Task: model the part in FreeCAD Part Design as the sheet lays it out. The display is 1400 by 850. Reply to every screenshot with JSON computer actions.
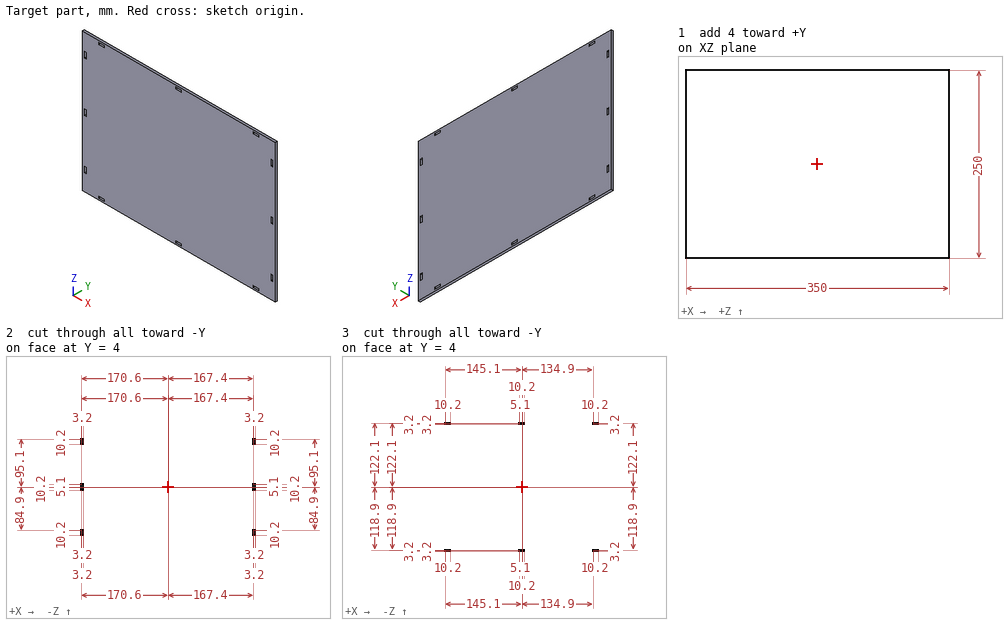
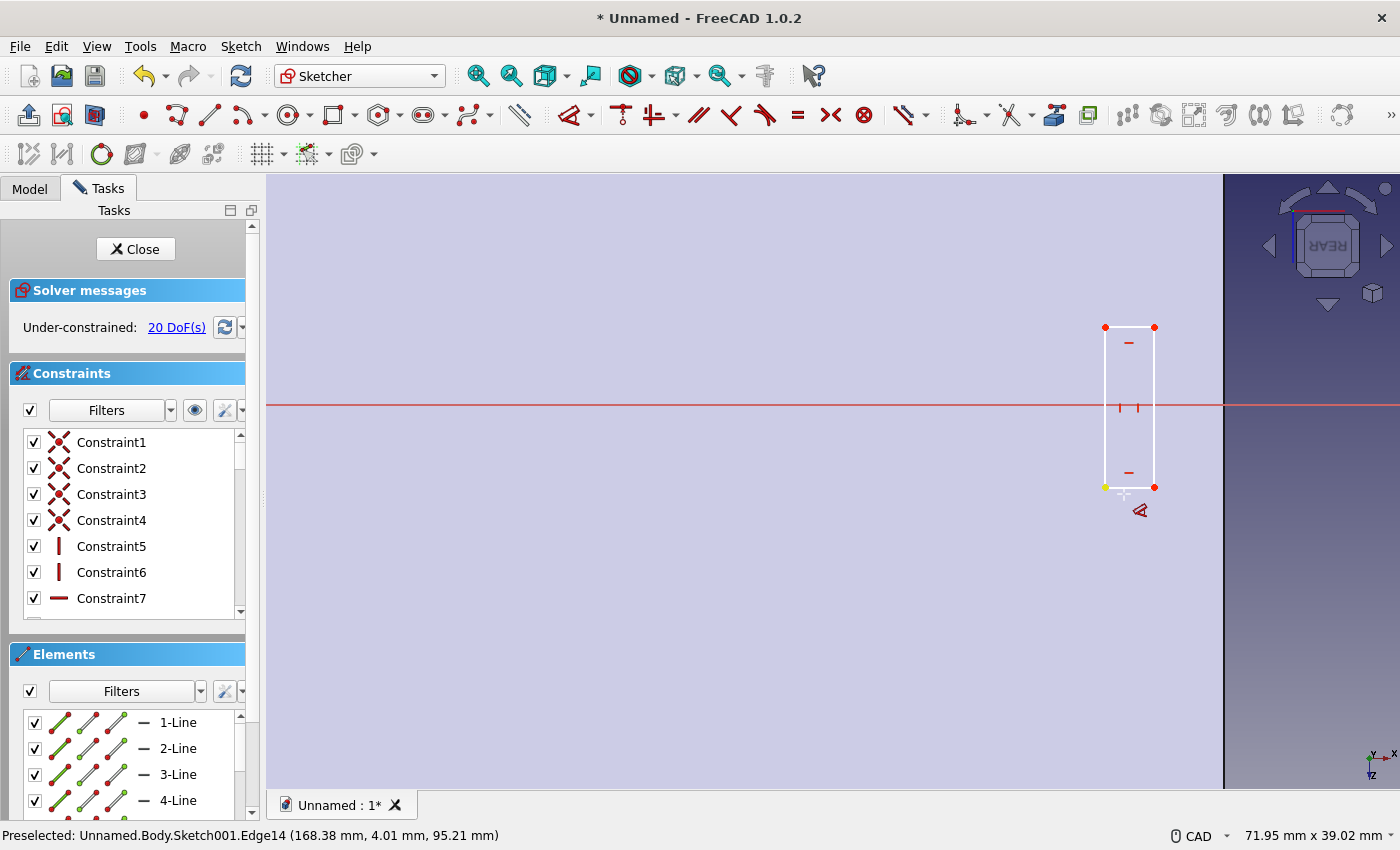
{"action": "left_click", "coordinate": [1120, 488]}
{"action": "left_click", "coordinate": [1130, 522]}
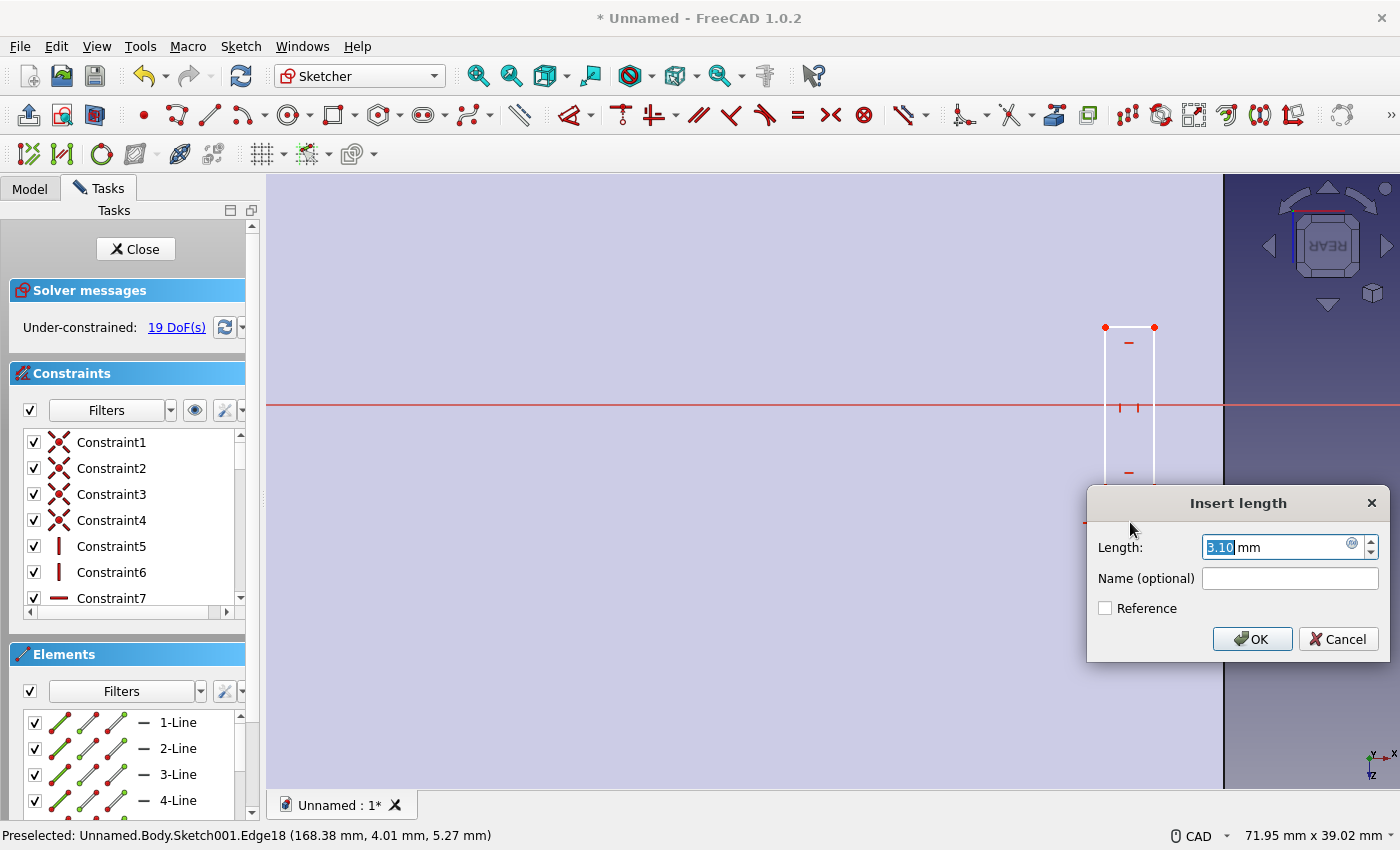
{"action": "type", "text": "3.2"}
{"action": "key", "text": "Return"}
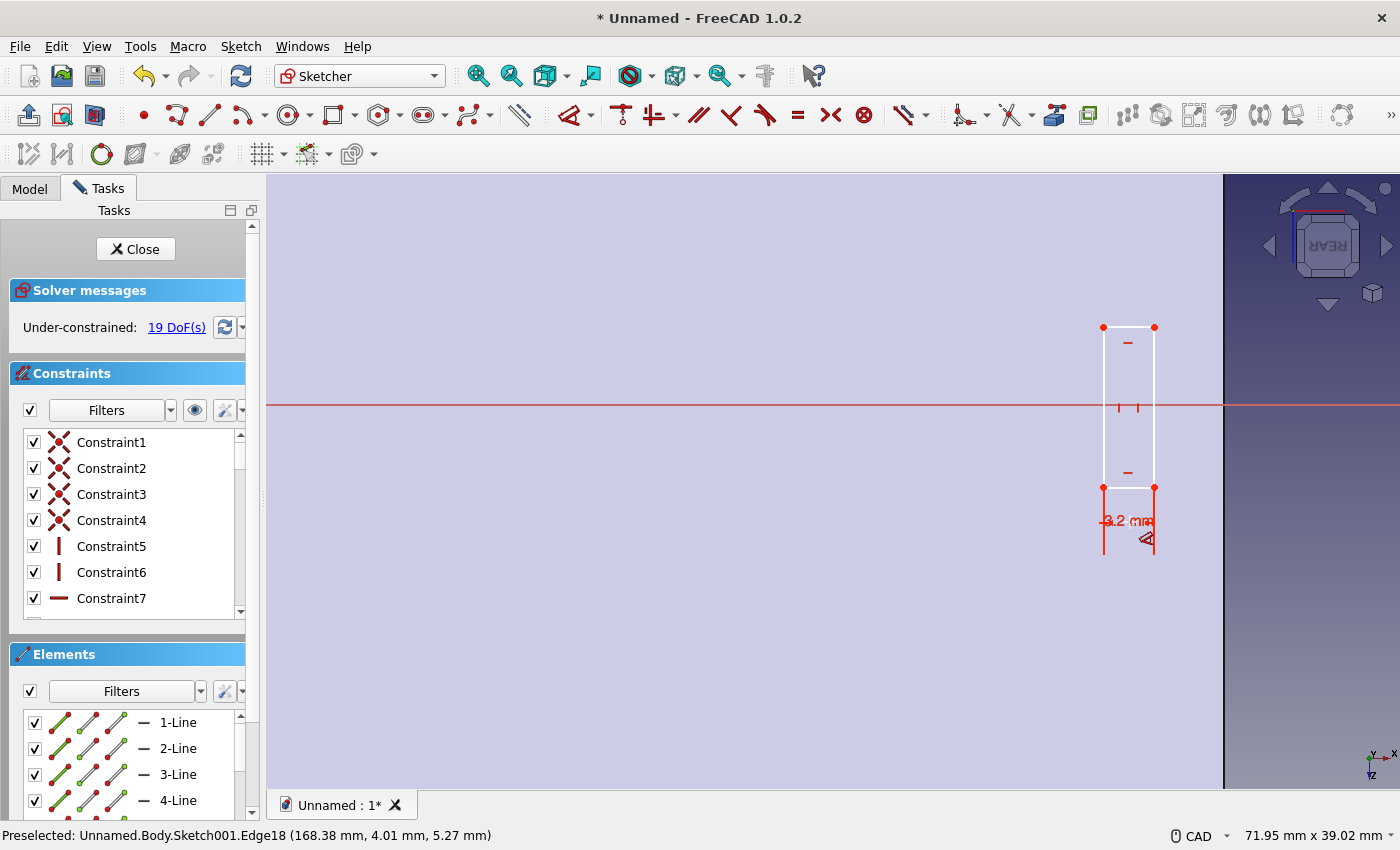
{"action": "scroll", "coordinate": [1124, 494], "scroll_direction": "down", "scroll_amount": 10}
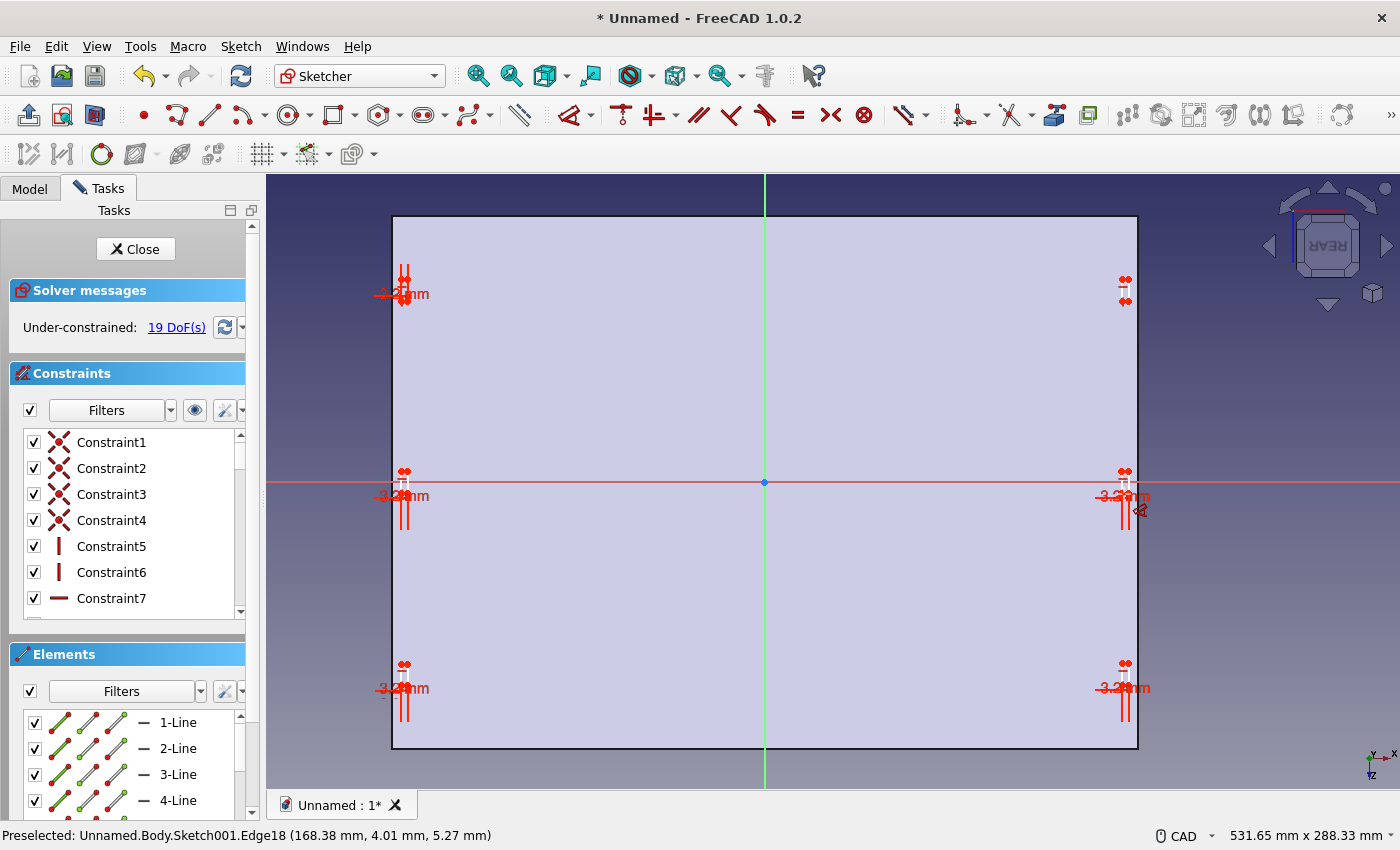
{"action": "scroll", "coordinate": [1124, 302], "scroll_direction": "up", "scroll_amount": 10}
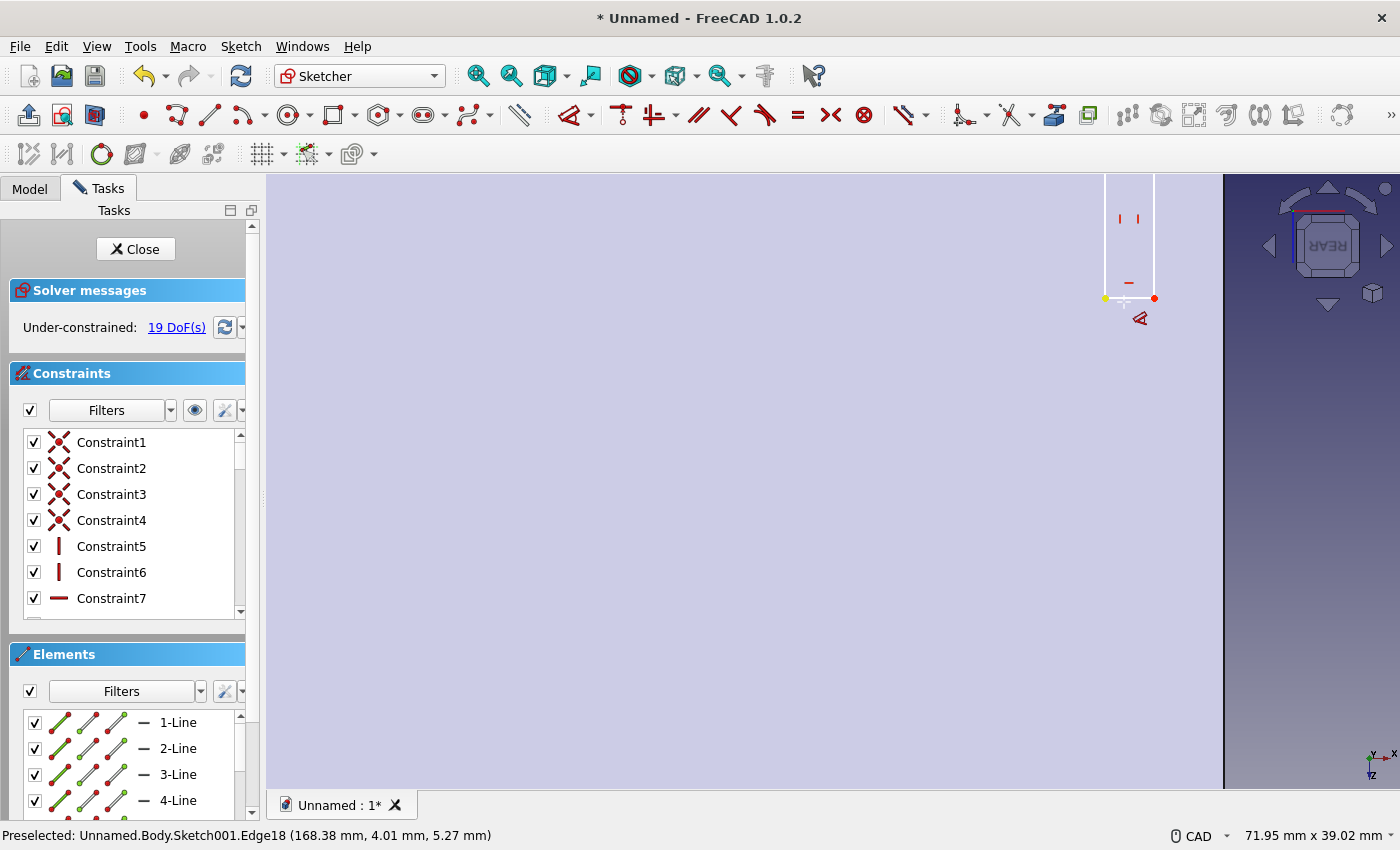
{"action": "left_click", "coordinate": [1120, 298]}
{"action": "left_click", "coordinate": [1130, 264]}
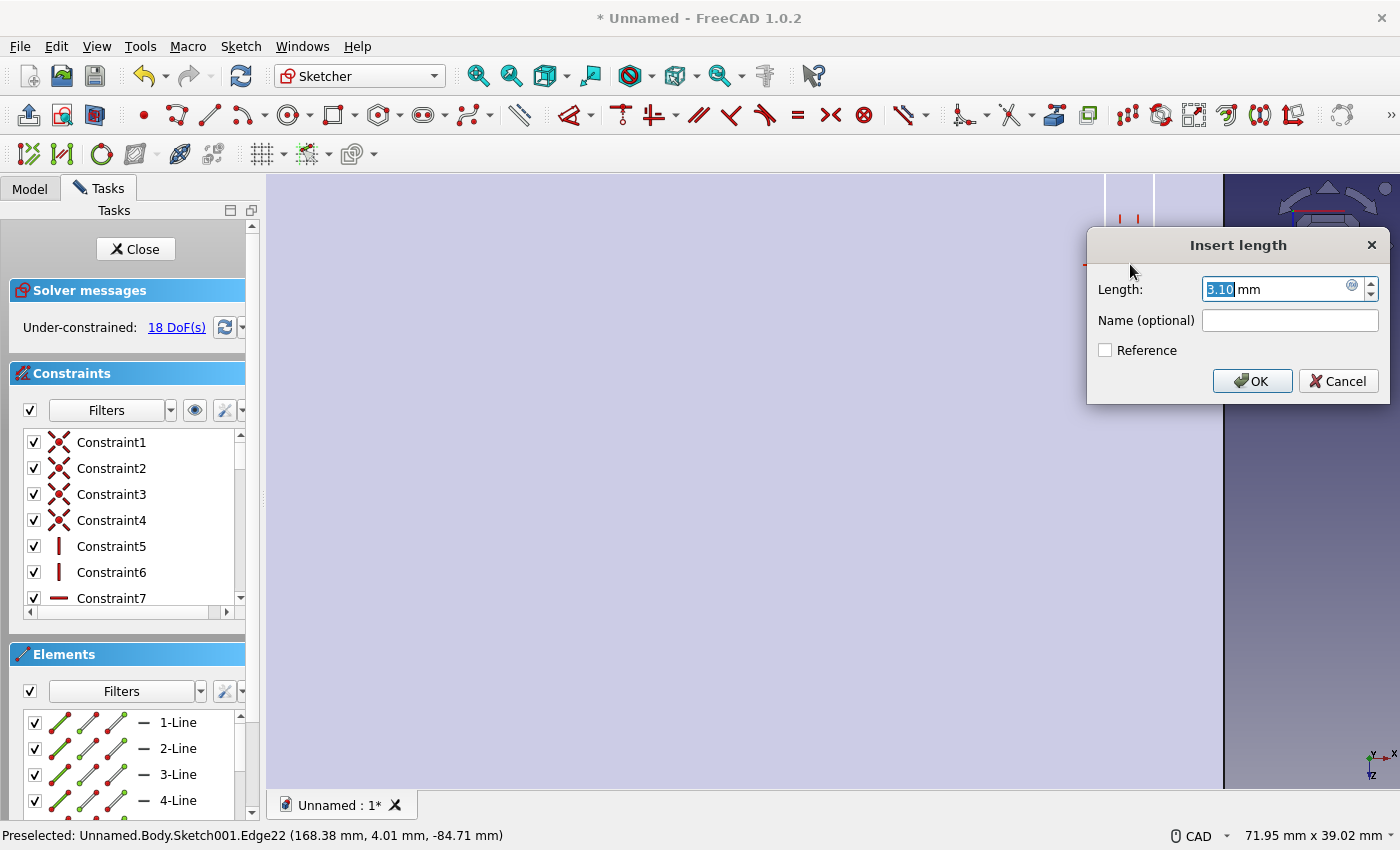
{"action": "type", "text": "3.2"}
{"action": "key", "text": "Return"}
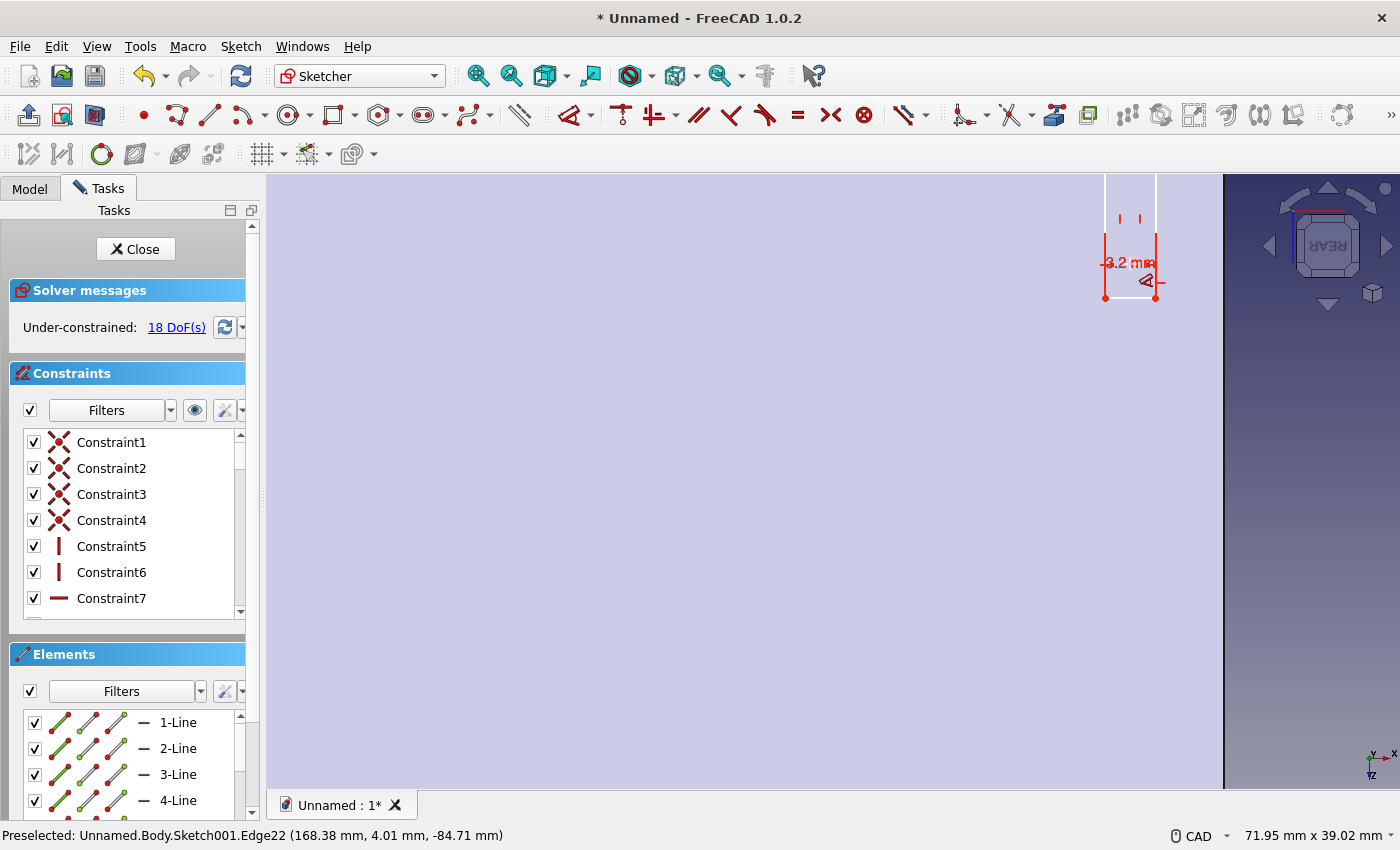
{"action": "scroll", "coordinate": [1124, 301], "scroll_direction": "down", "scroll_amount": 10}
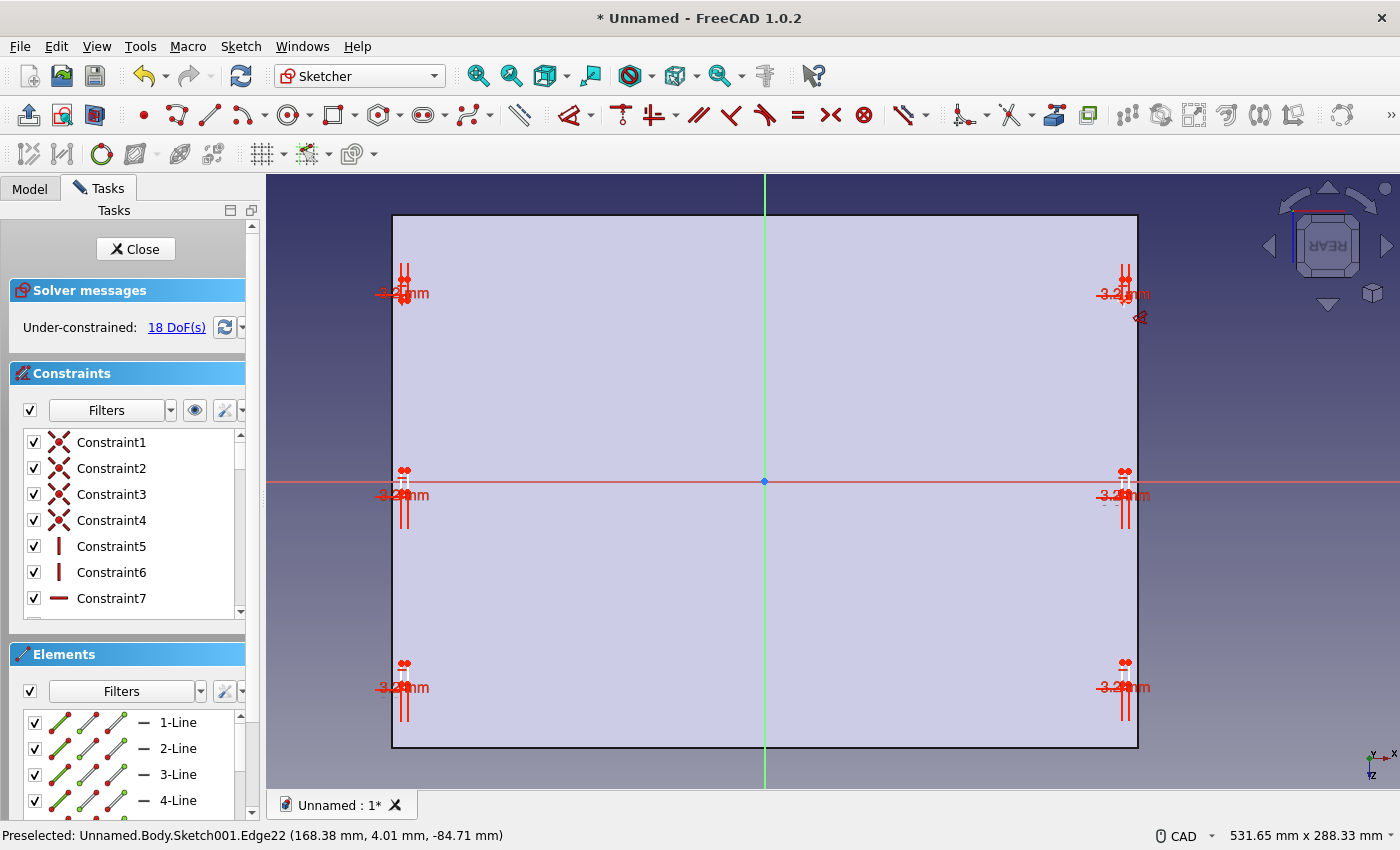
{"action": "scroll", "coordinate": [401, 286], "scroll_direction": "up", "scroll_amount": 4}